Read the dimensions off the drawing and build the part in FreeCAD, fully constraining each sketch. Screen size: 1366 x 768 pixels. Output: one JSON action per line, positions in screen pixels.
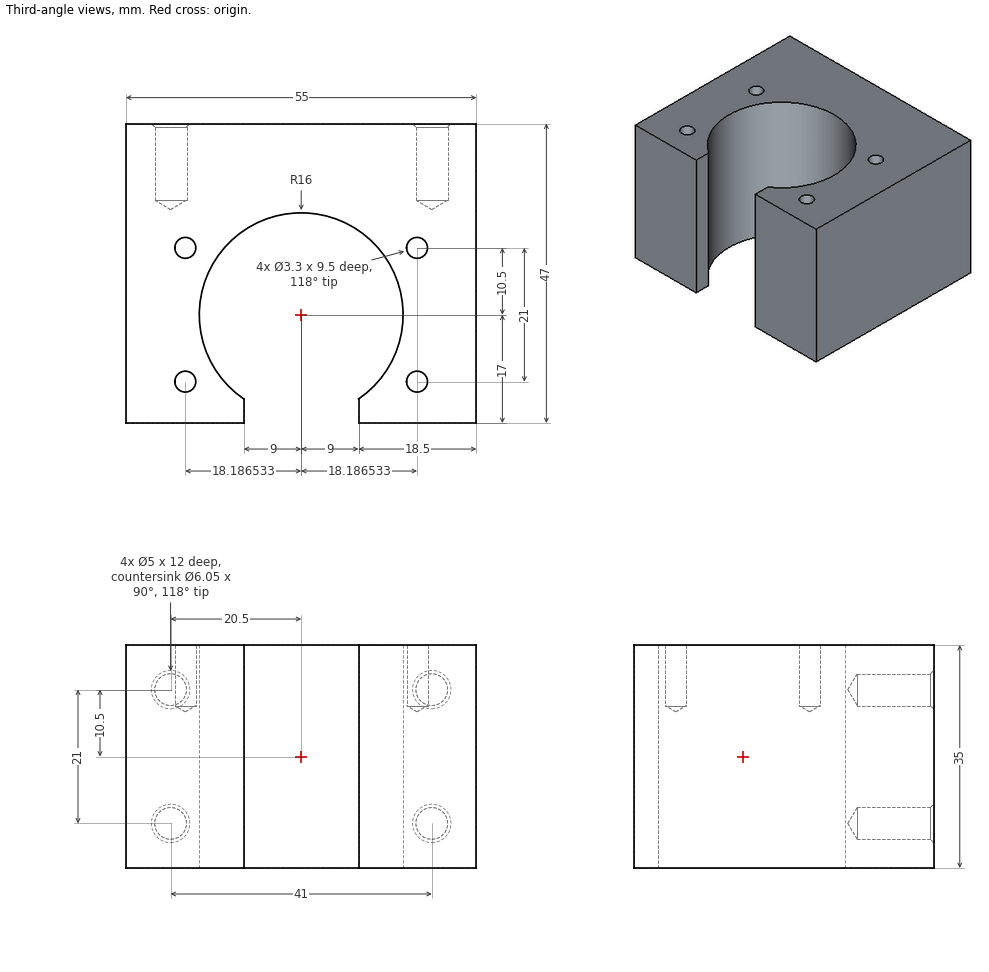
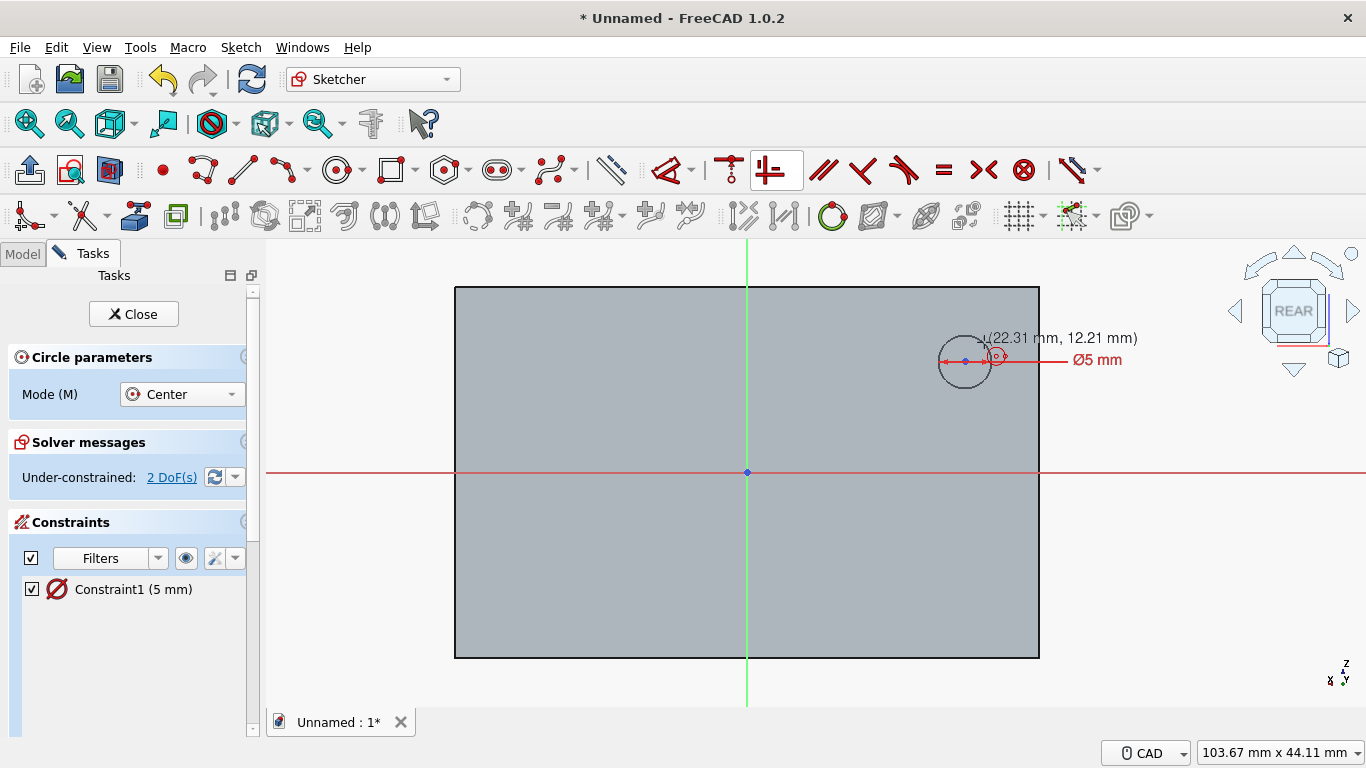
{"action": "left_click", "coordinate": [965, 584]}
{"action": "mouse_move", "coordinate": [984, 565]}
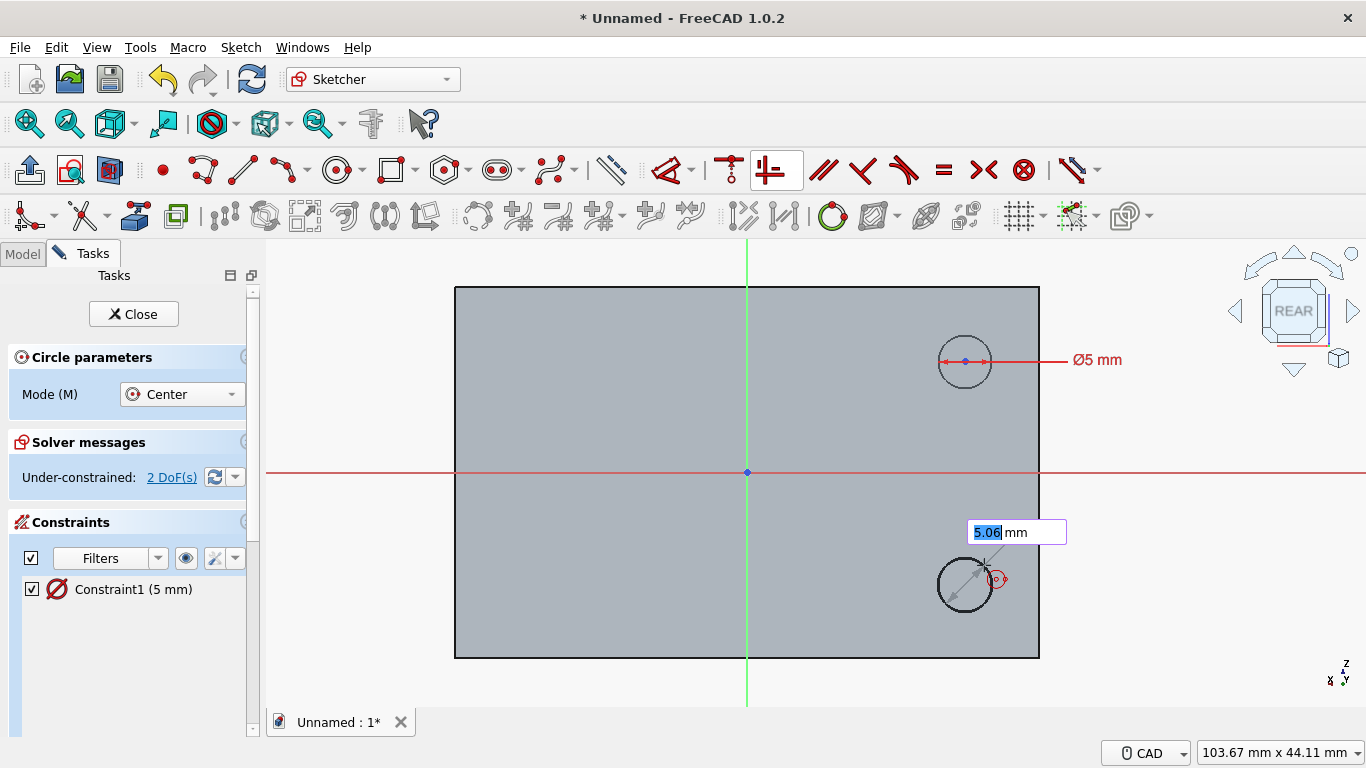
{"action": "type", "text": "5"}
{"action": "key", "text": "Return"}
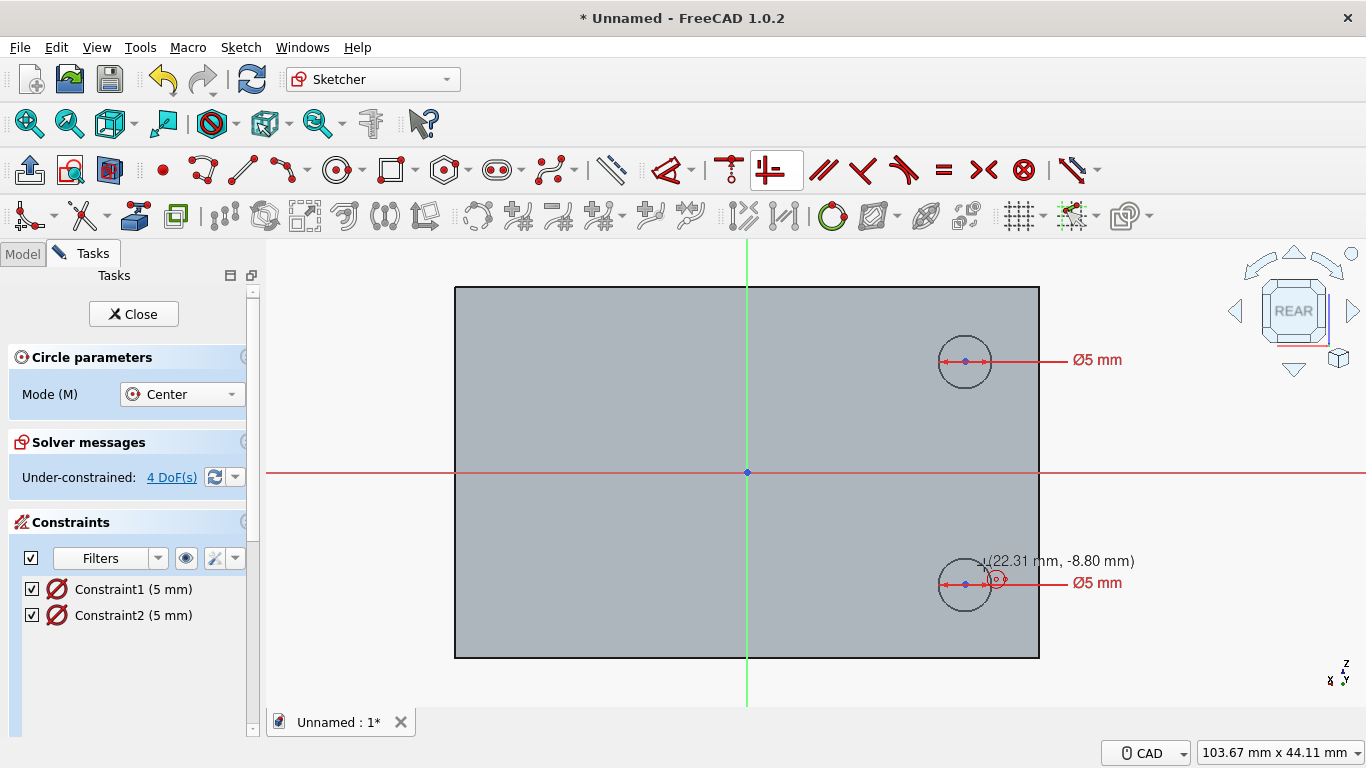
{"action": "left_click", "coordinate": [530, 584]}
{"action": "mouse_move", "coordinate": [549, 565]}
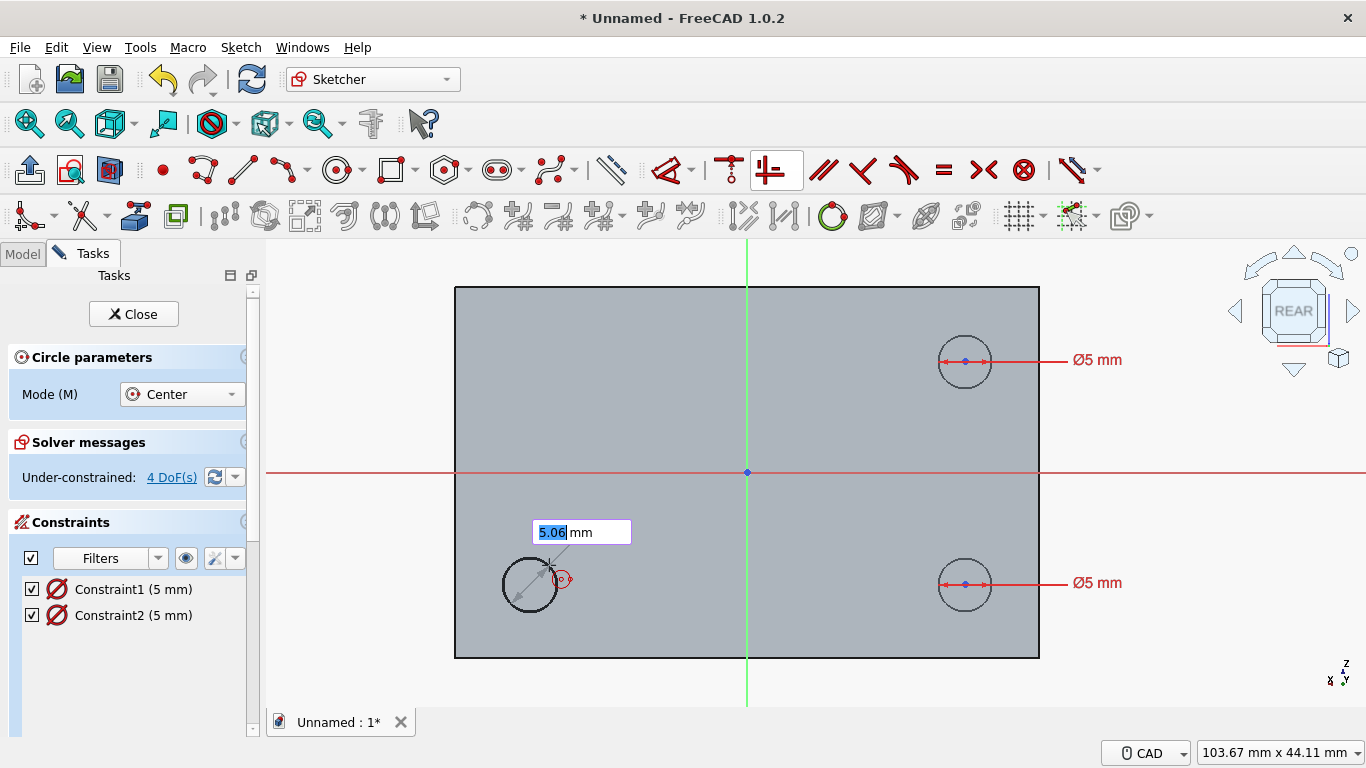
{"action": "type", "text": "5"}
{"action": "key", "text": "Return"}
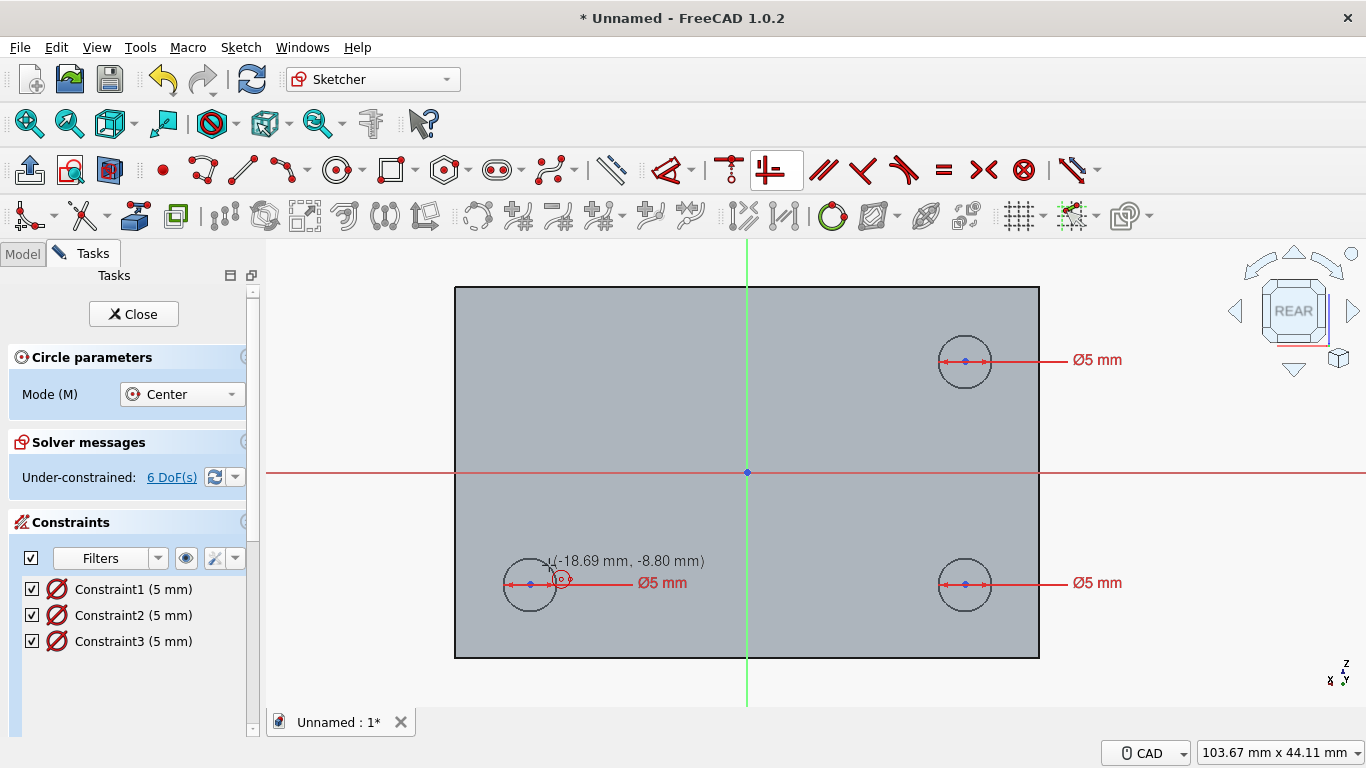
{"action": "left_click", "coordinate": [530, 361]}
{"action": "mouse_move", "coordinate": [549, 342]}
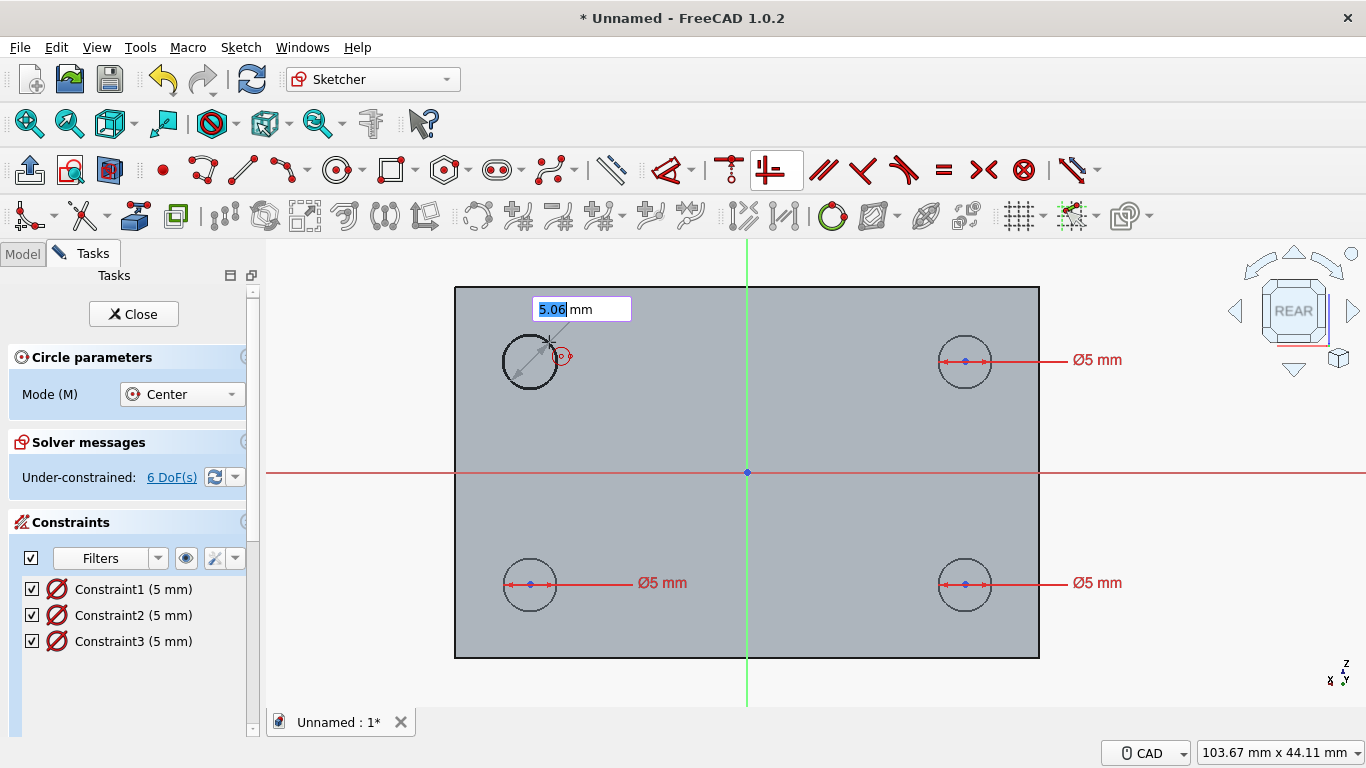
{"action": "type", "text": "5"}
{"action": "key", "text": "Return"}
{"action": "key", "text": "Escape"}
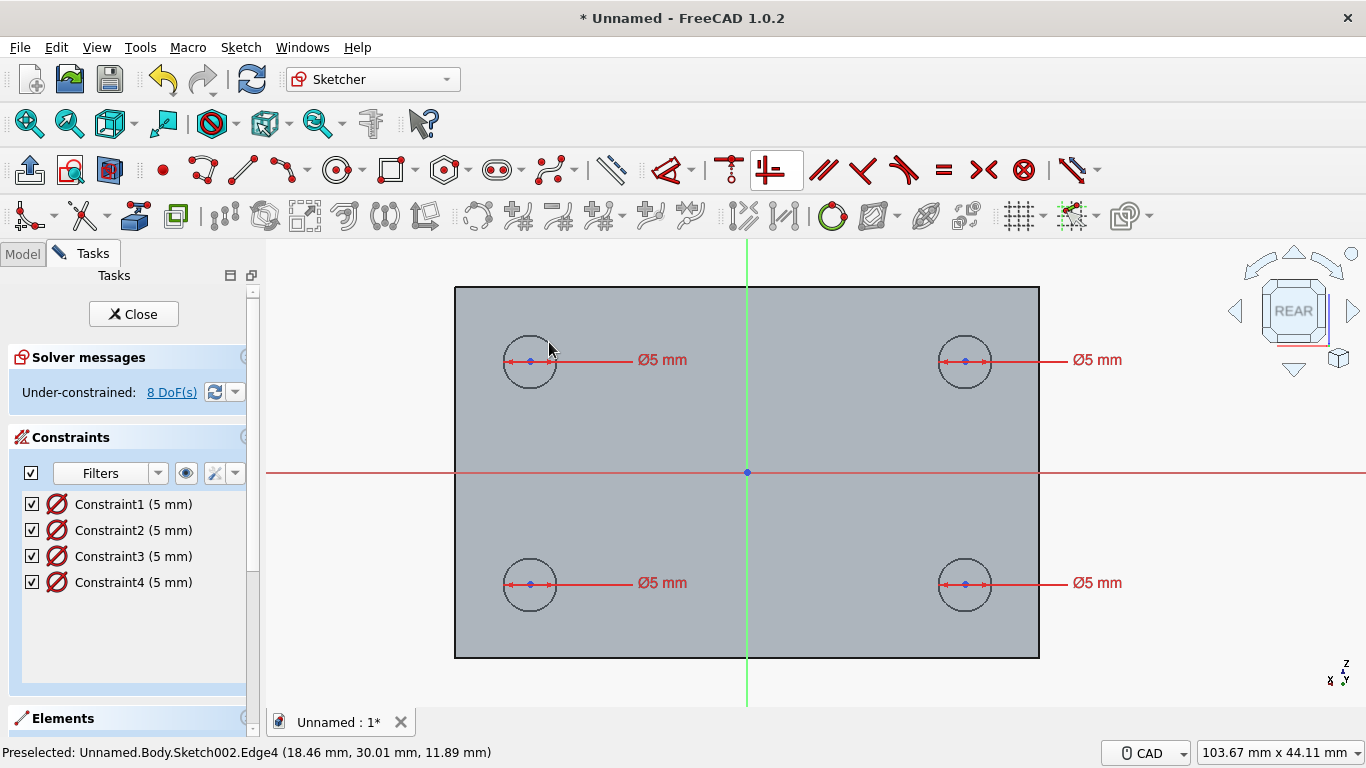
{"action": "key", "text": "d"}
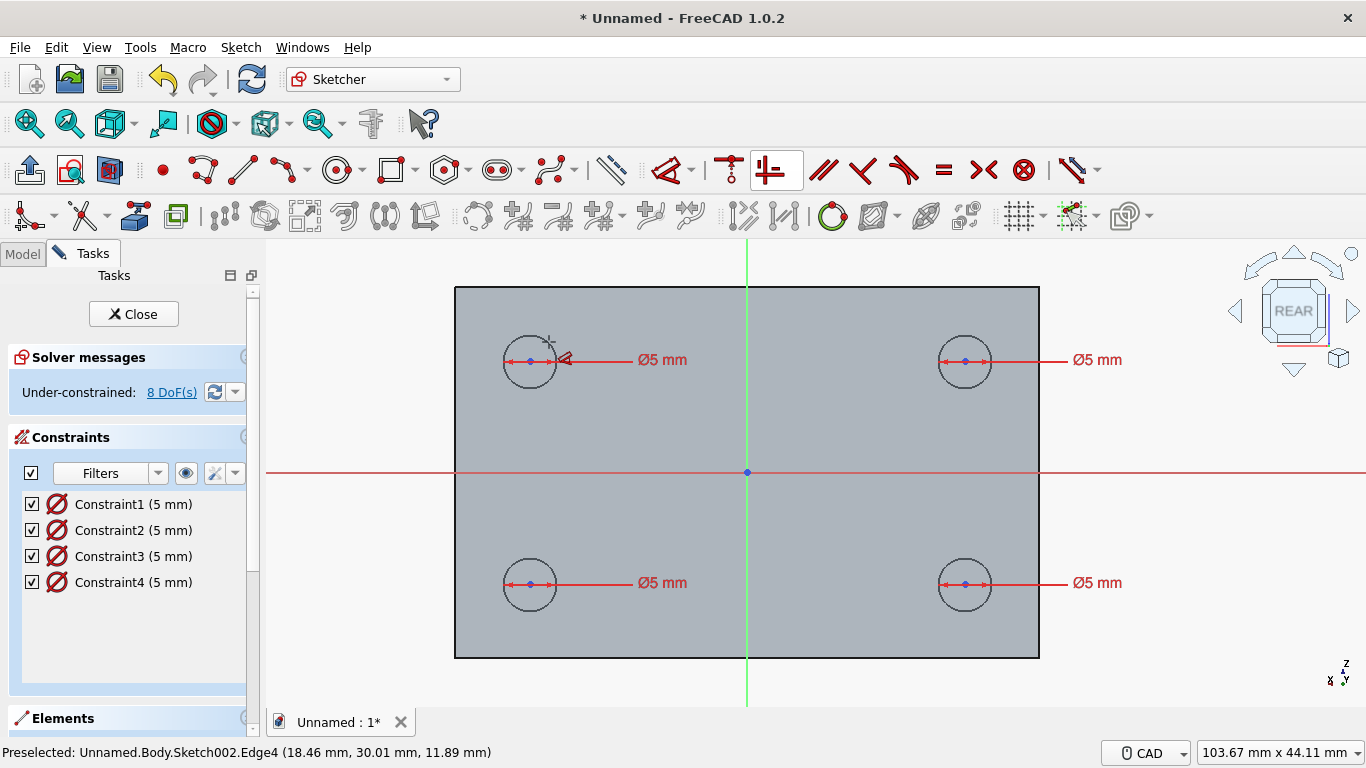
{"action": "left_click", "coordinate": [965, 362]}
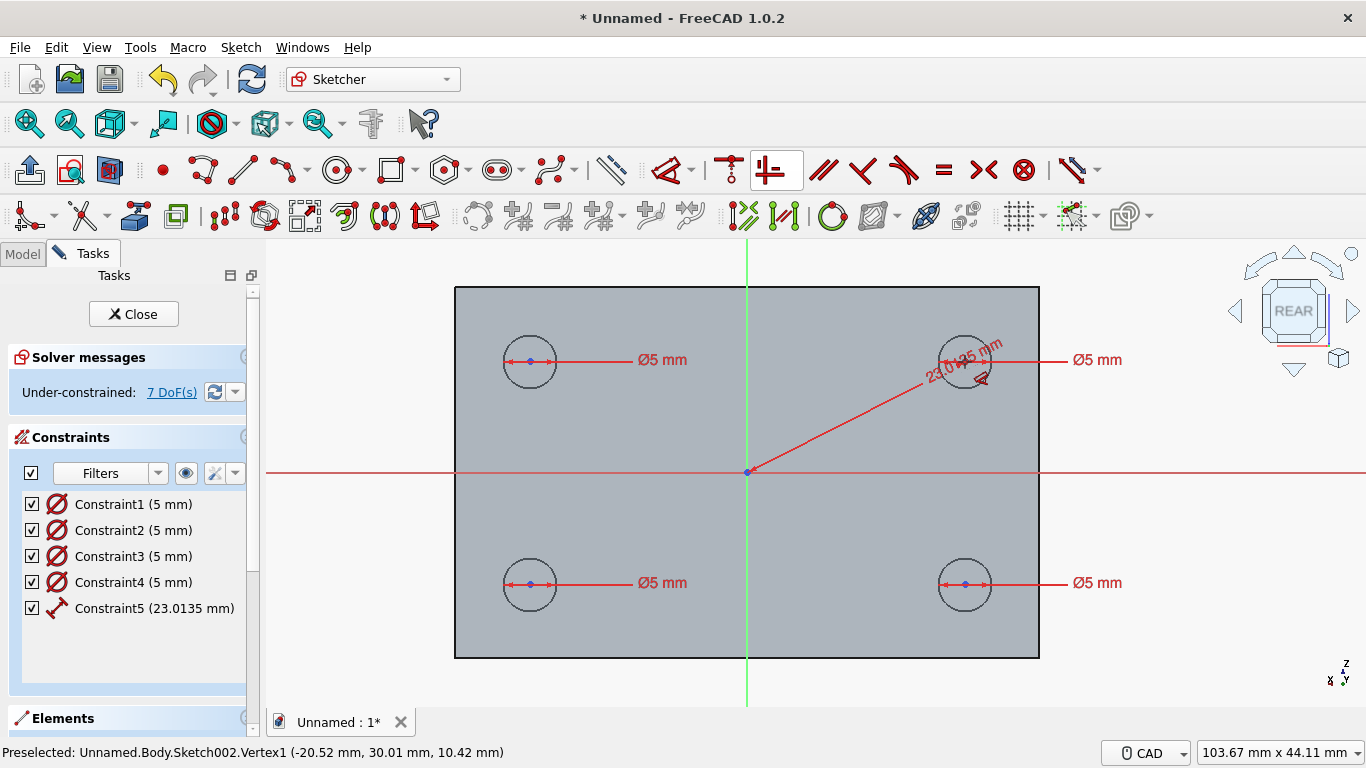
{"action": "left_click", "coordinate": [965, 585]}
{"action": "left_click", "coordinate": [999, 422]}